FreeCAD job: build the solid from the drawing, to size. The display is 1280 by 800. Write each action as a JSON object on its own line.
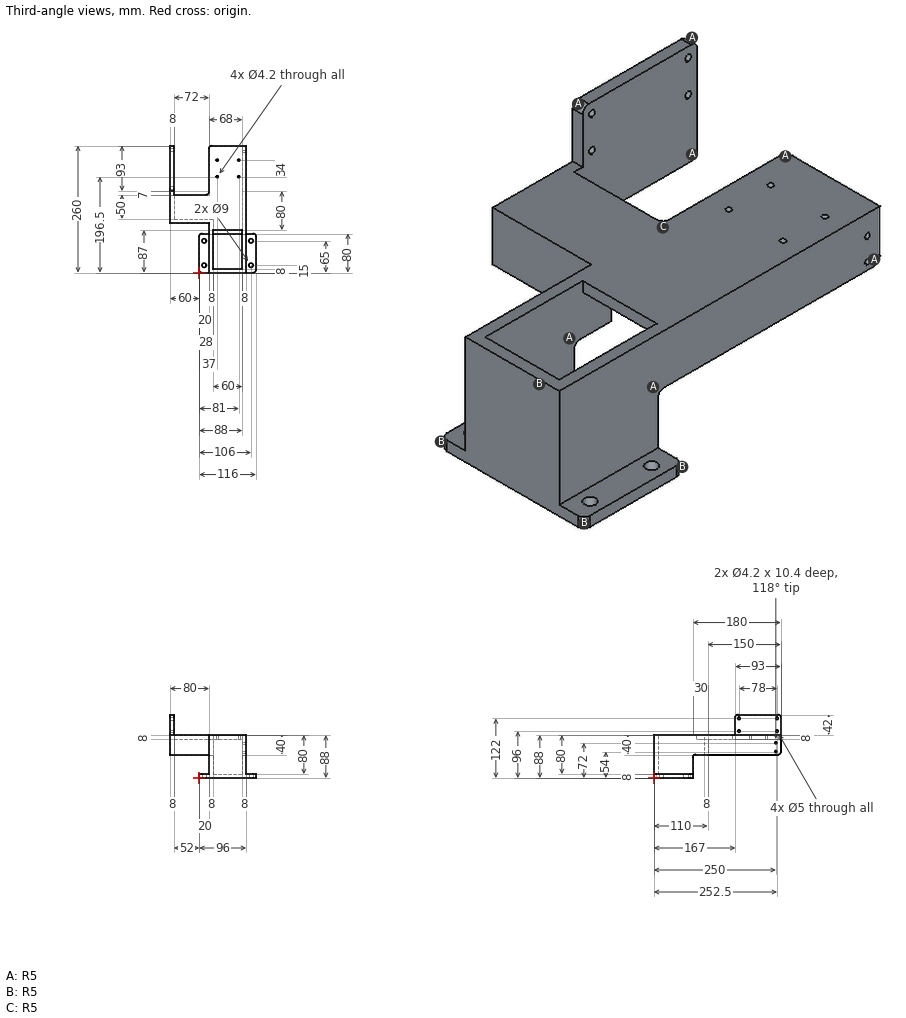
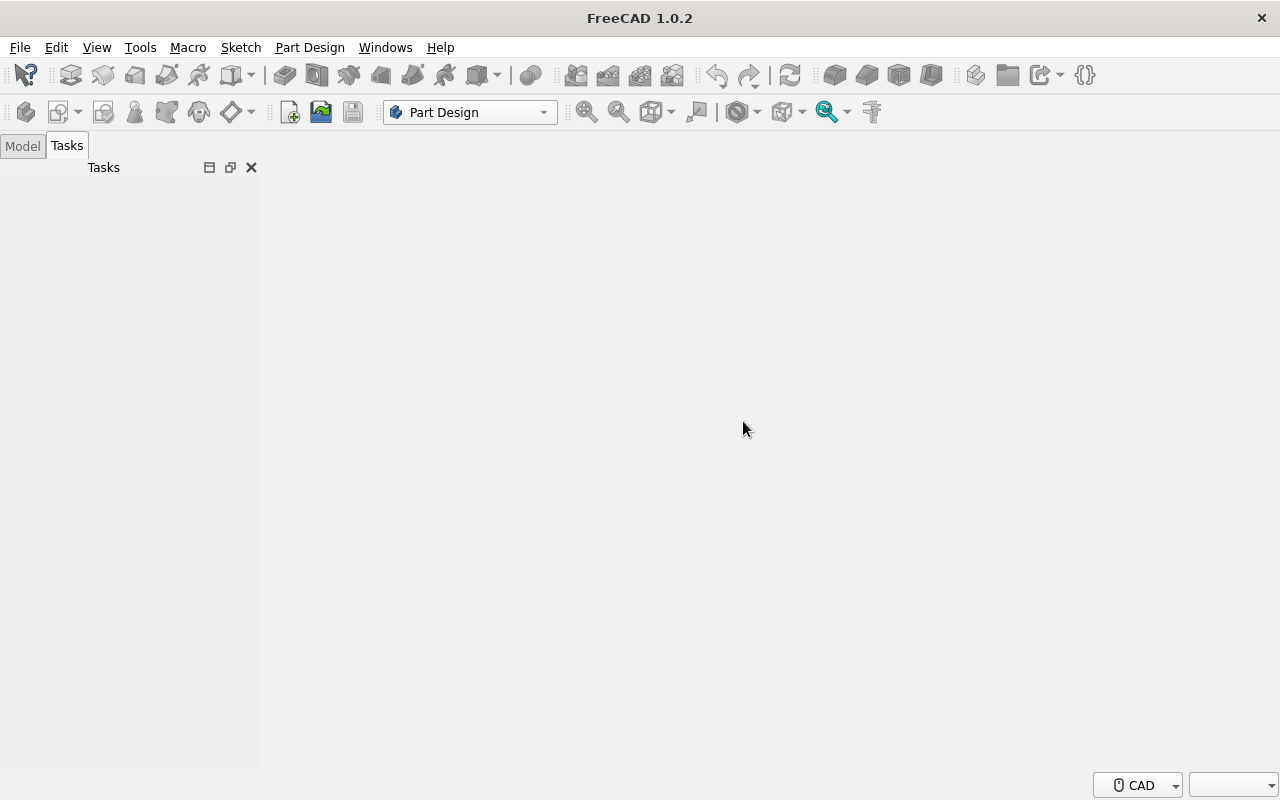
{"action": "left_click", "coordinate": [290, 112]}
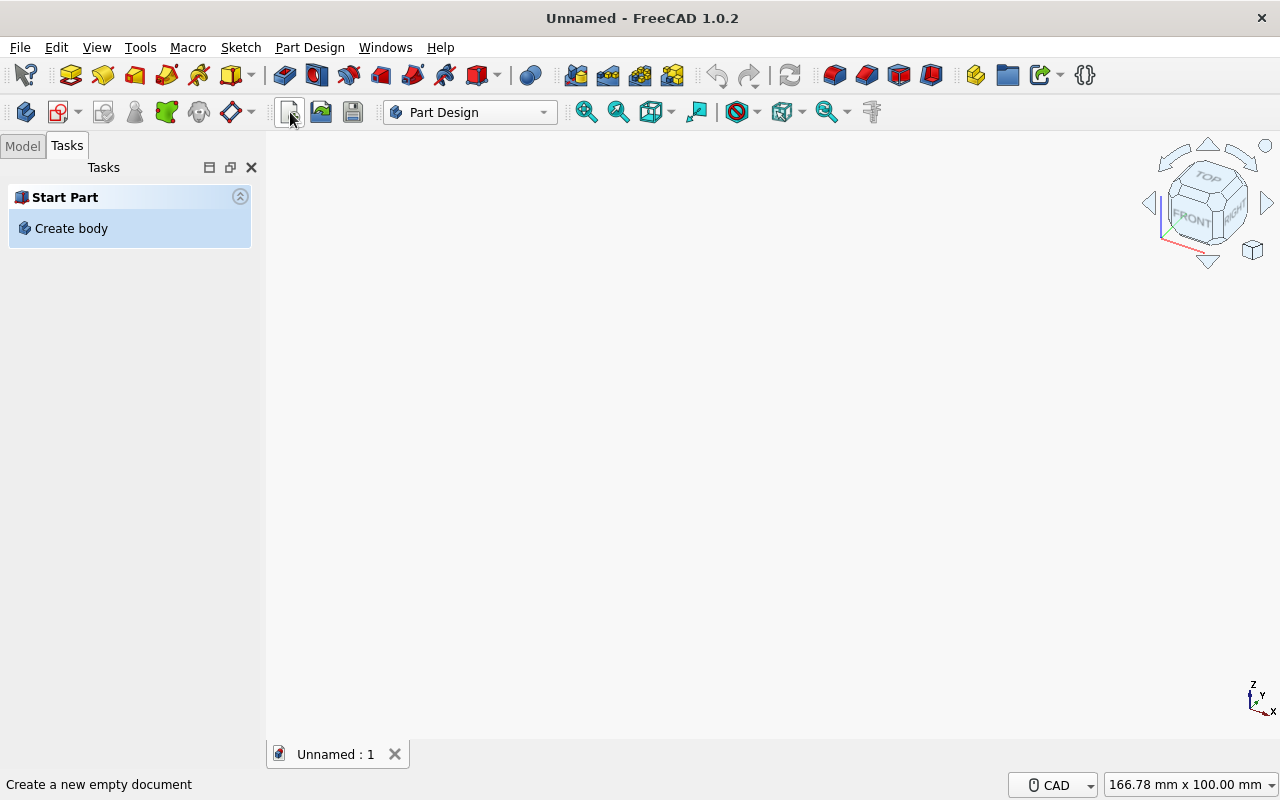
{"action": "left_click", "coordinate": [58, 112]}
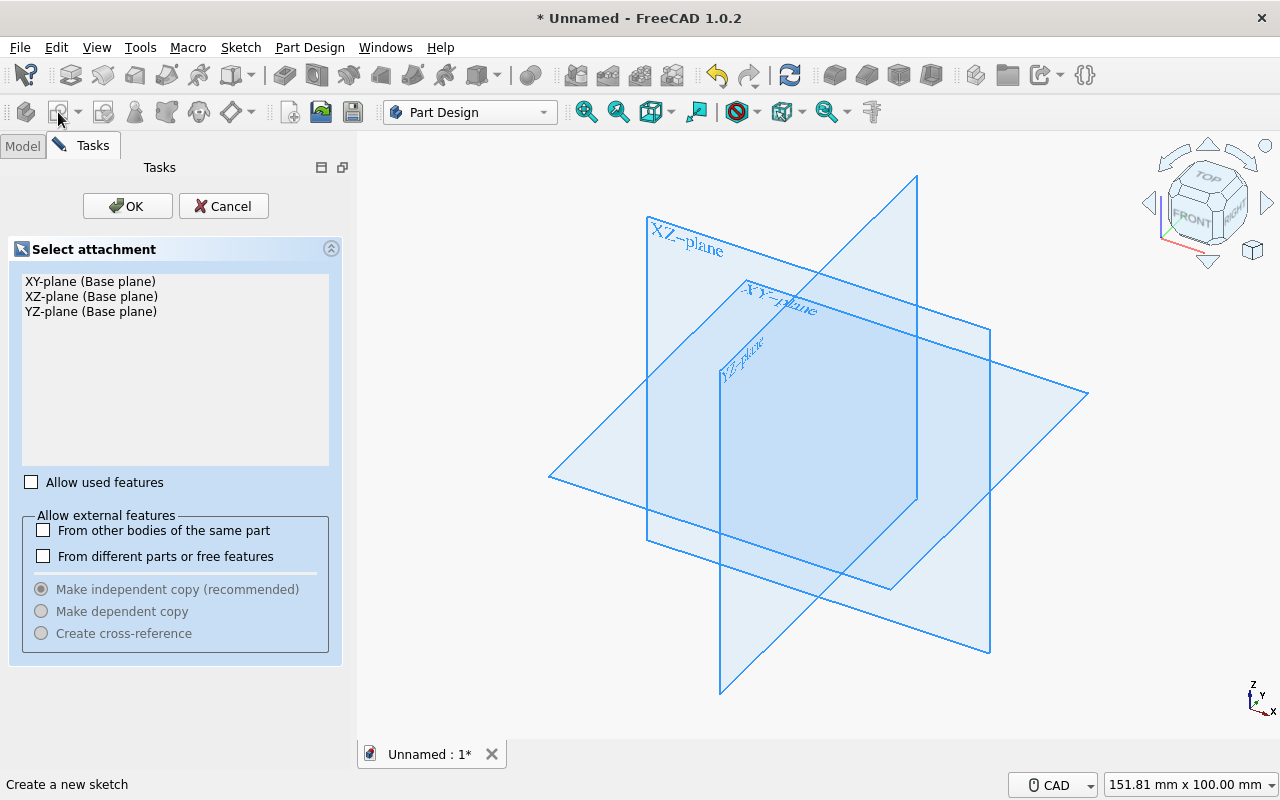
{"action": "left_click", "coordinate": [82, 282]}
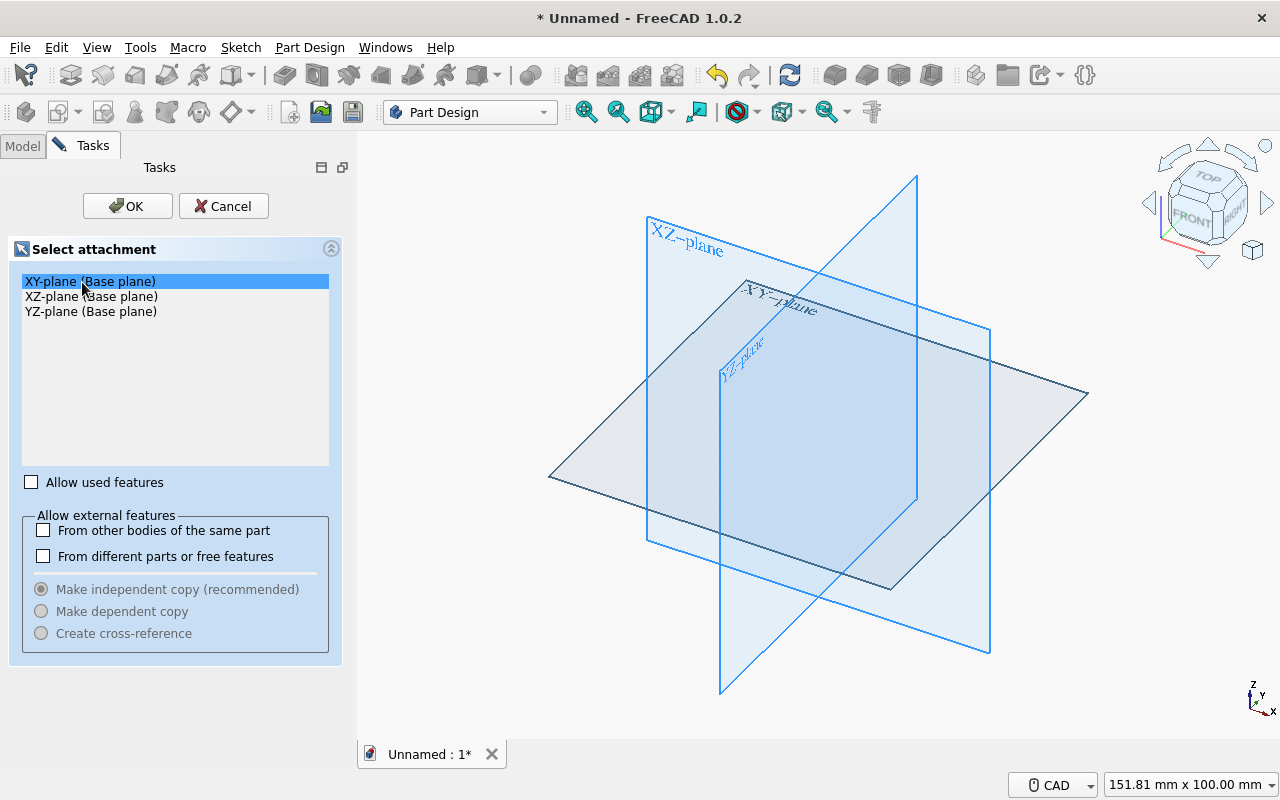
{"action": "left_click", "coordinate": [128, 206]}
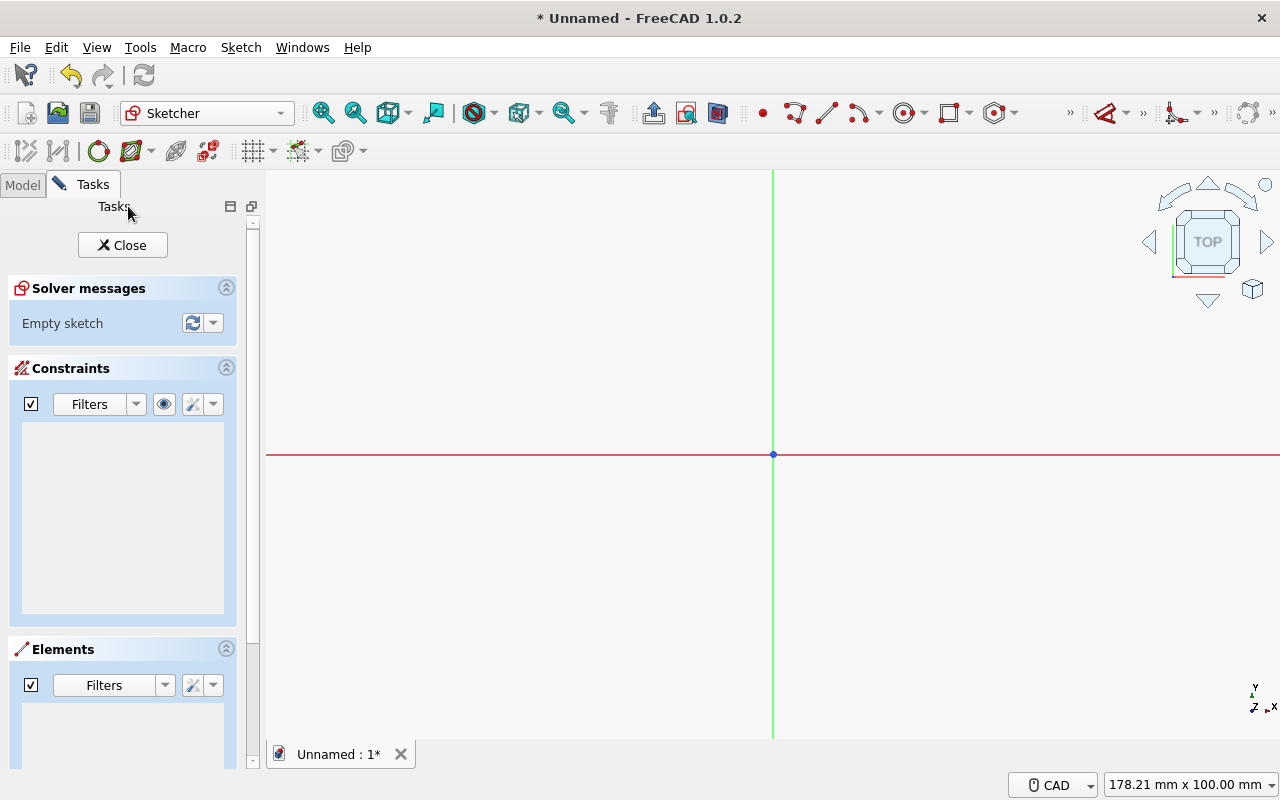
{"action": "scroll", "coordinate": [294, 711], "scroll_direction": "down", "scroll_amount": 2}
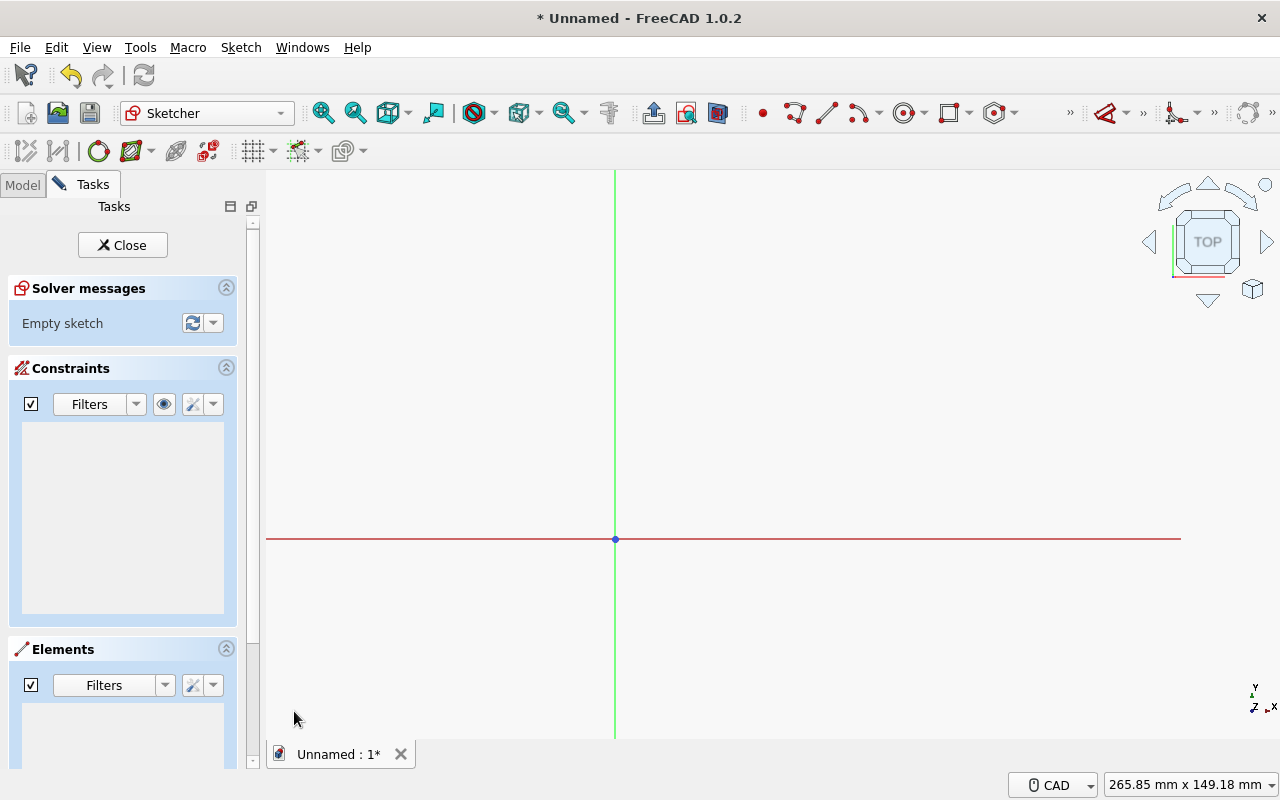
{"action": "left_click", "coordinate": [950, 114]}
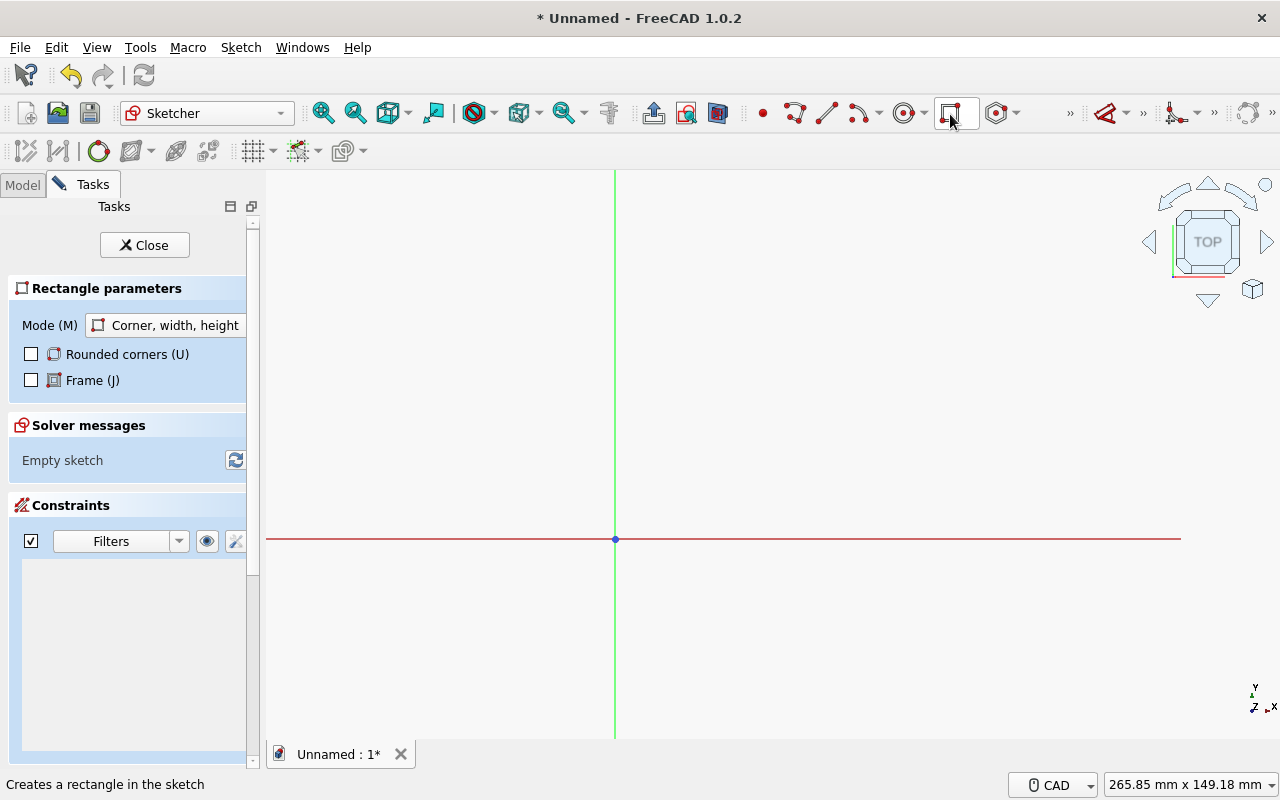
{"action": "left_click", "coordinate": [615, 539]}
{"action": "left_click", "coordinate": [1058, 234]}
{"action": "key", "text": "Escape"}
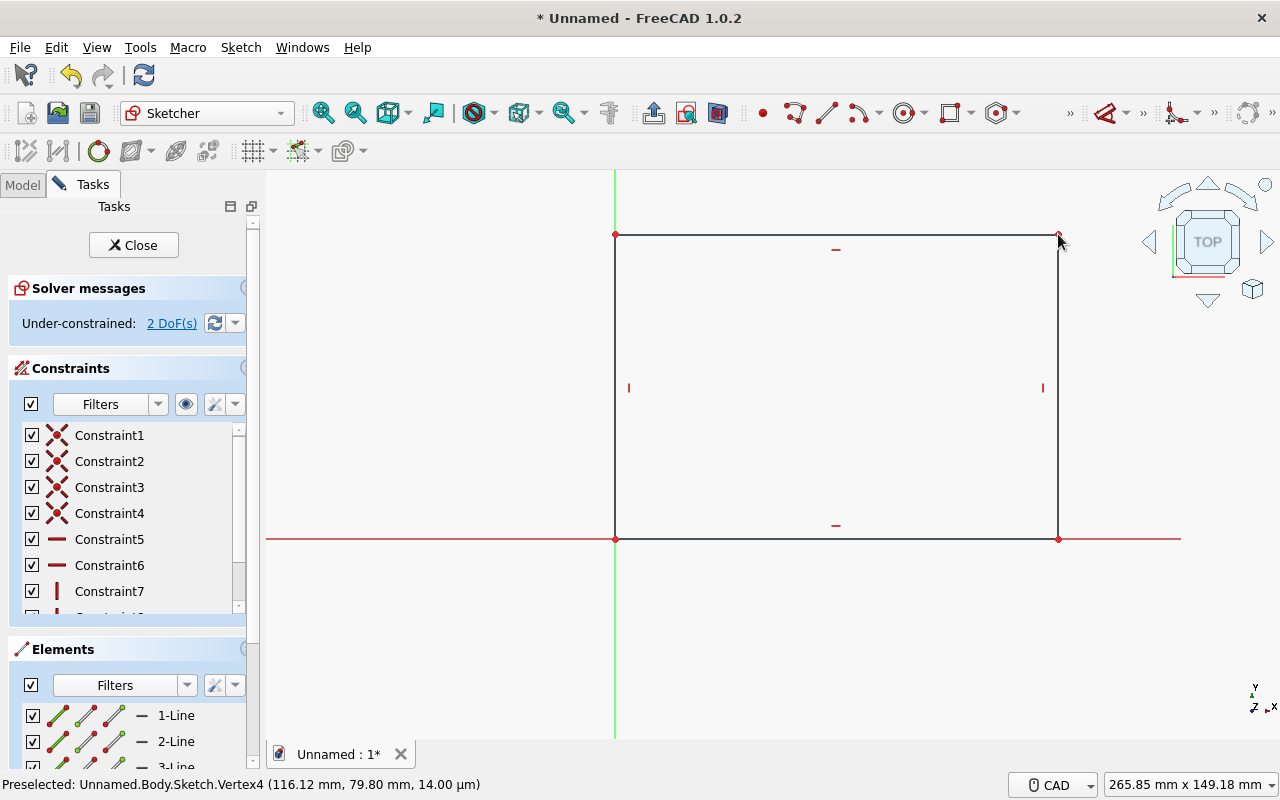
{"action": "left_click", "coordinate": [1058, 448]}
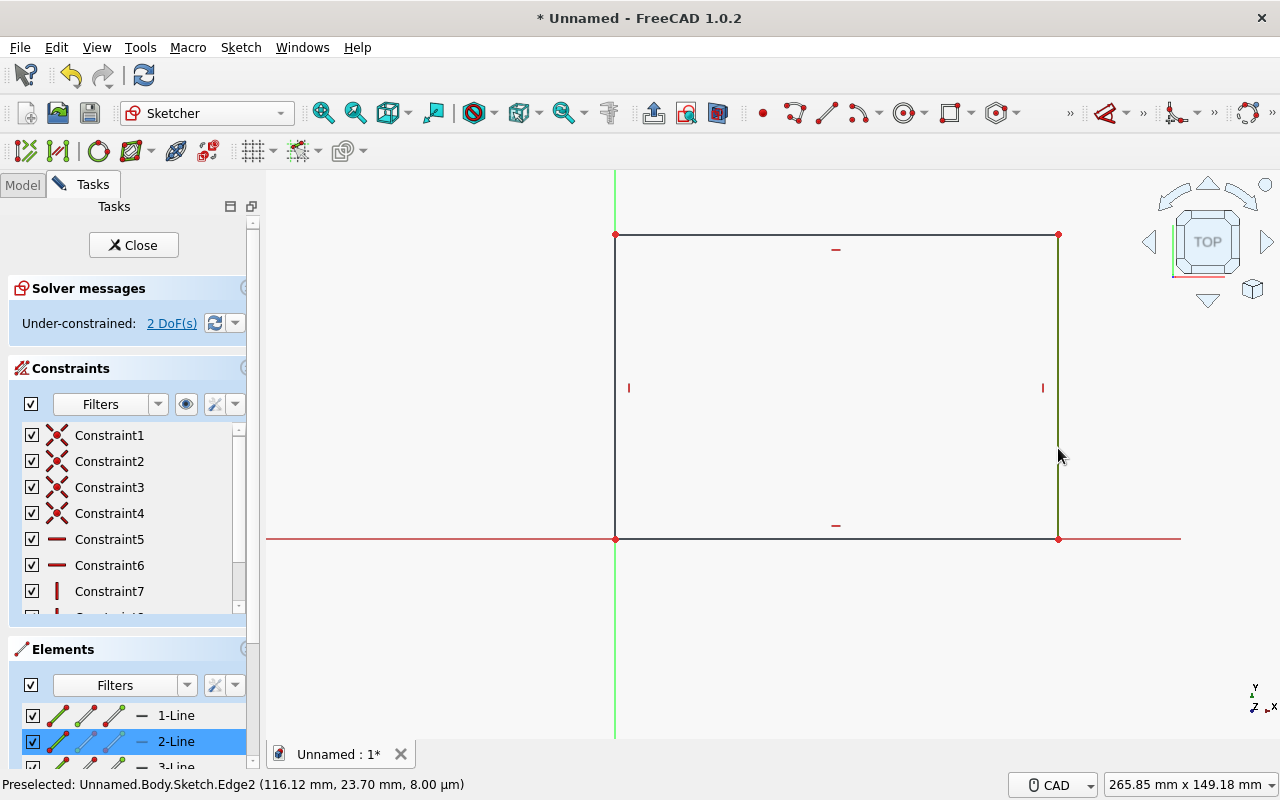
{"action": "left_click", "coordinate": [1128, 114]}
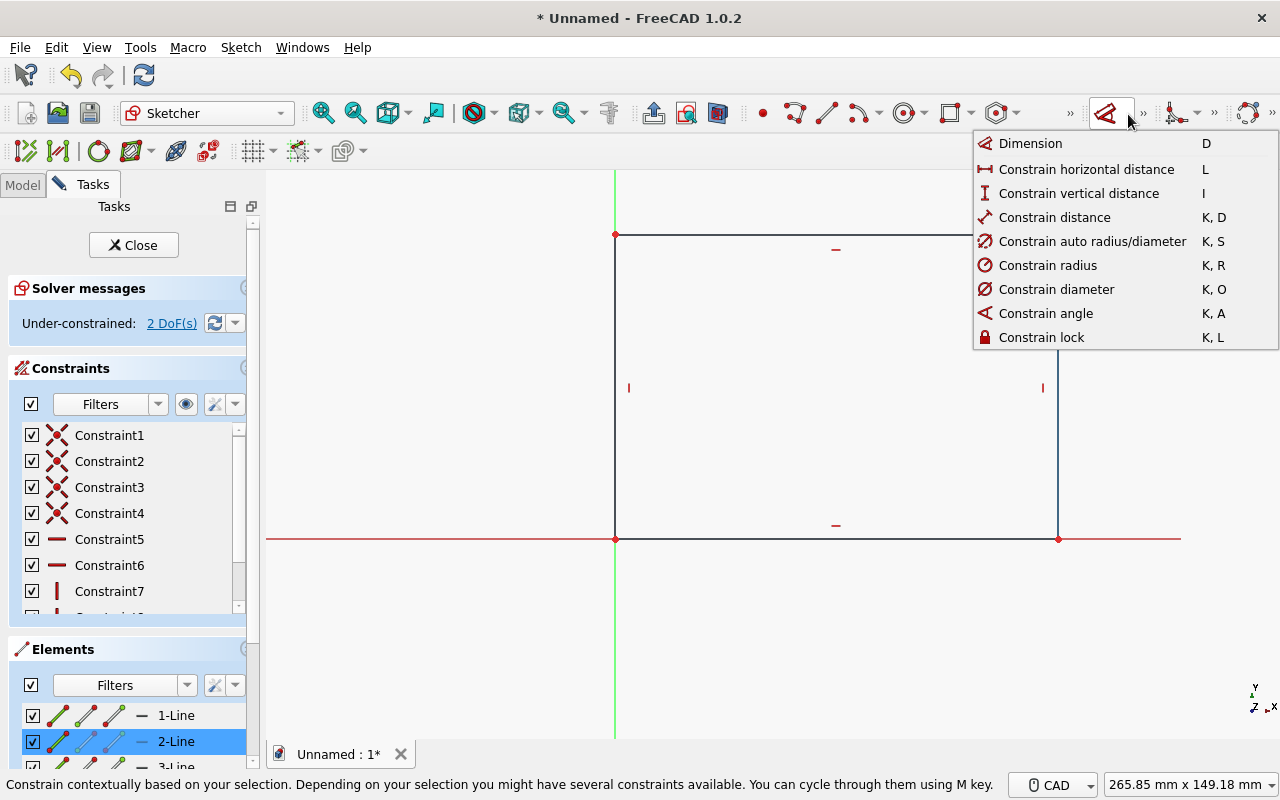
{"action": "left_click", "coordinate": [1126, 193]}